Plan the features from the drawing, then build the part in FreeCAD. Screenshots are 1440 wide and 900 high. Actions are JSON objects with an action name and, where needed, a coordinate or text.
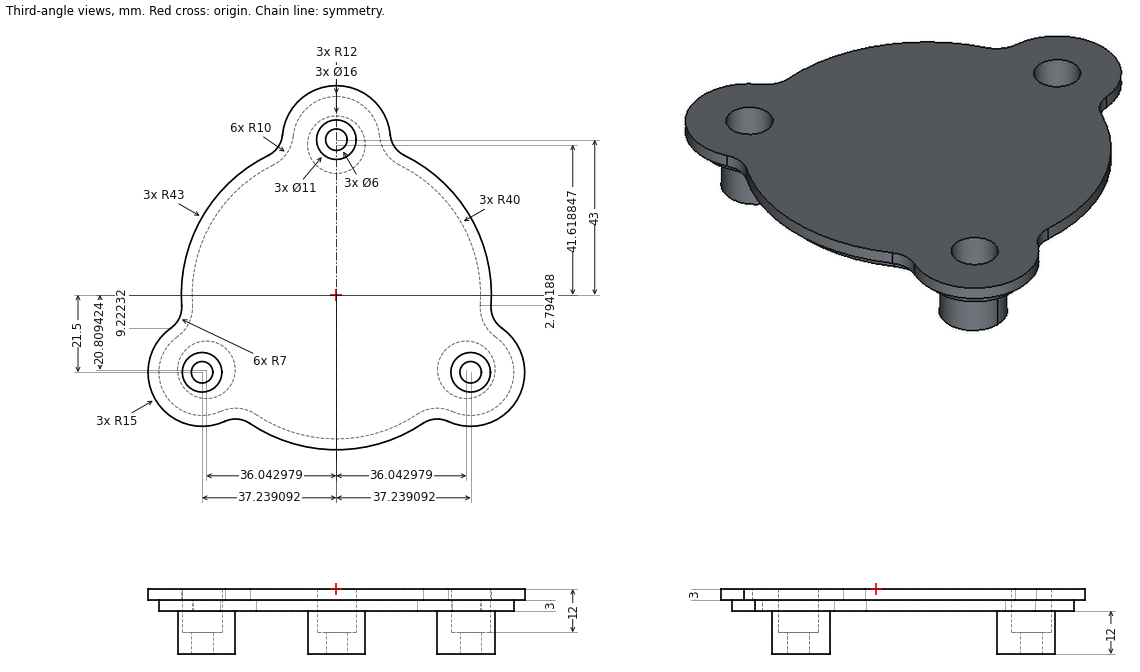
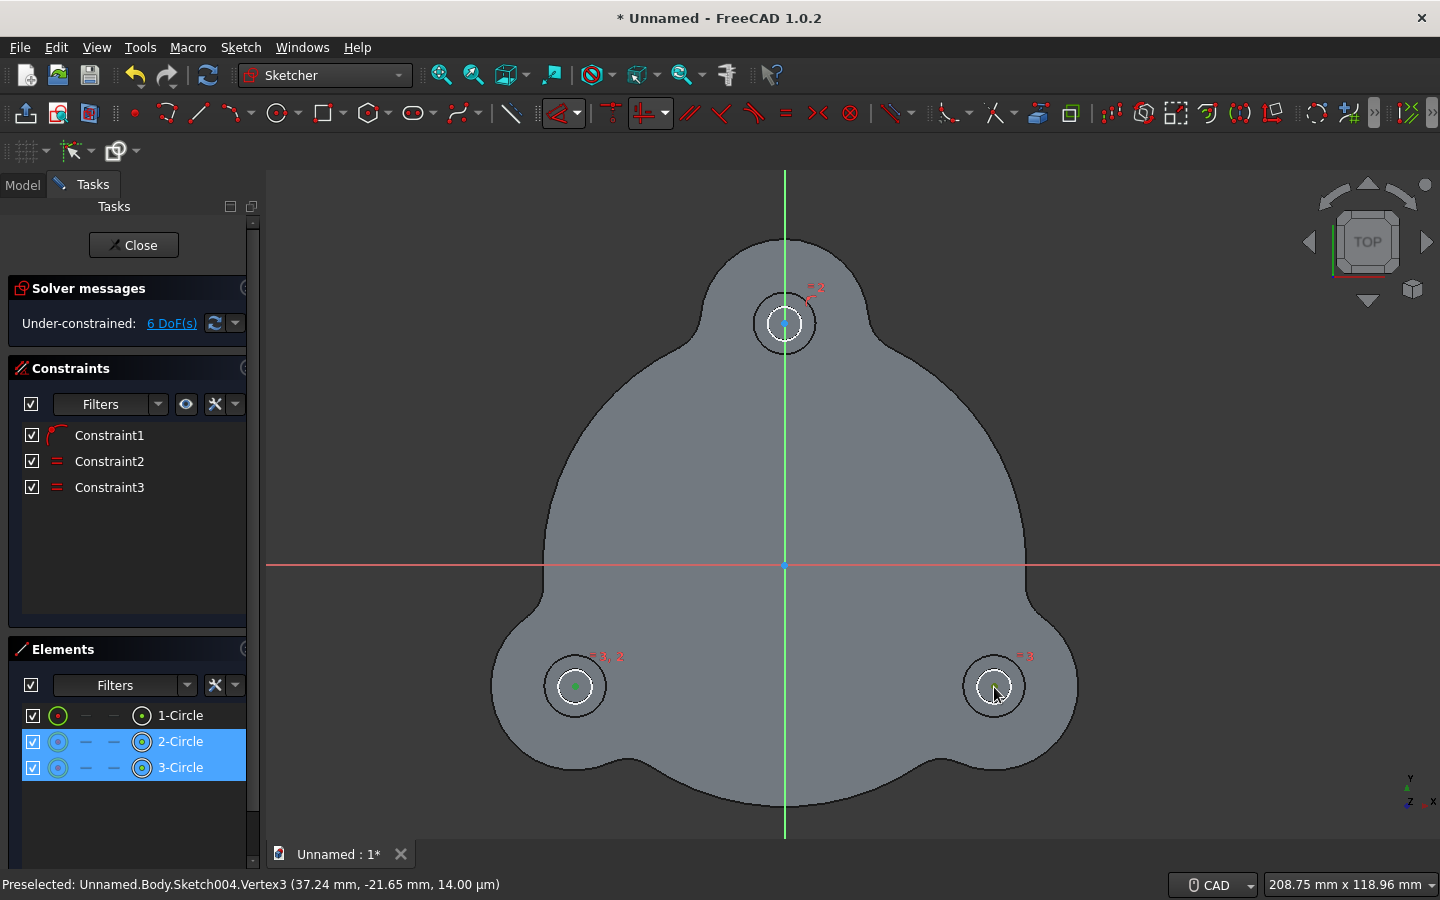
{"action": "key", "text": "h"}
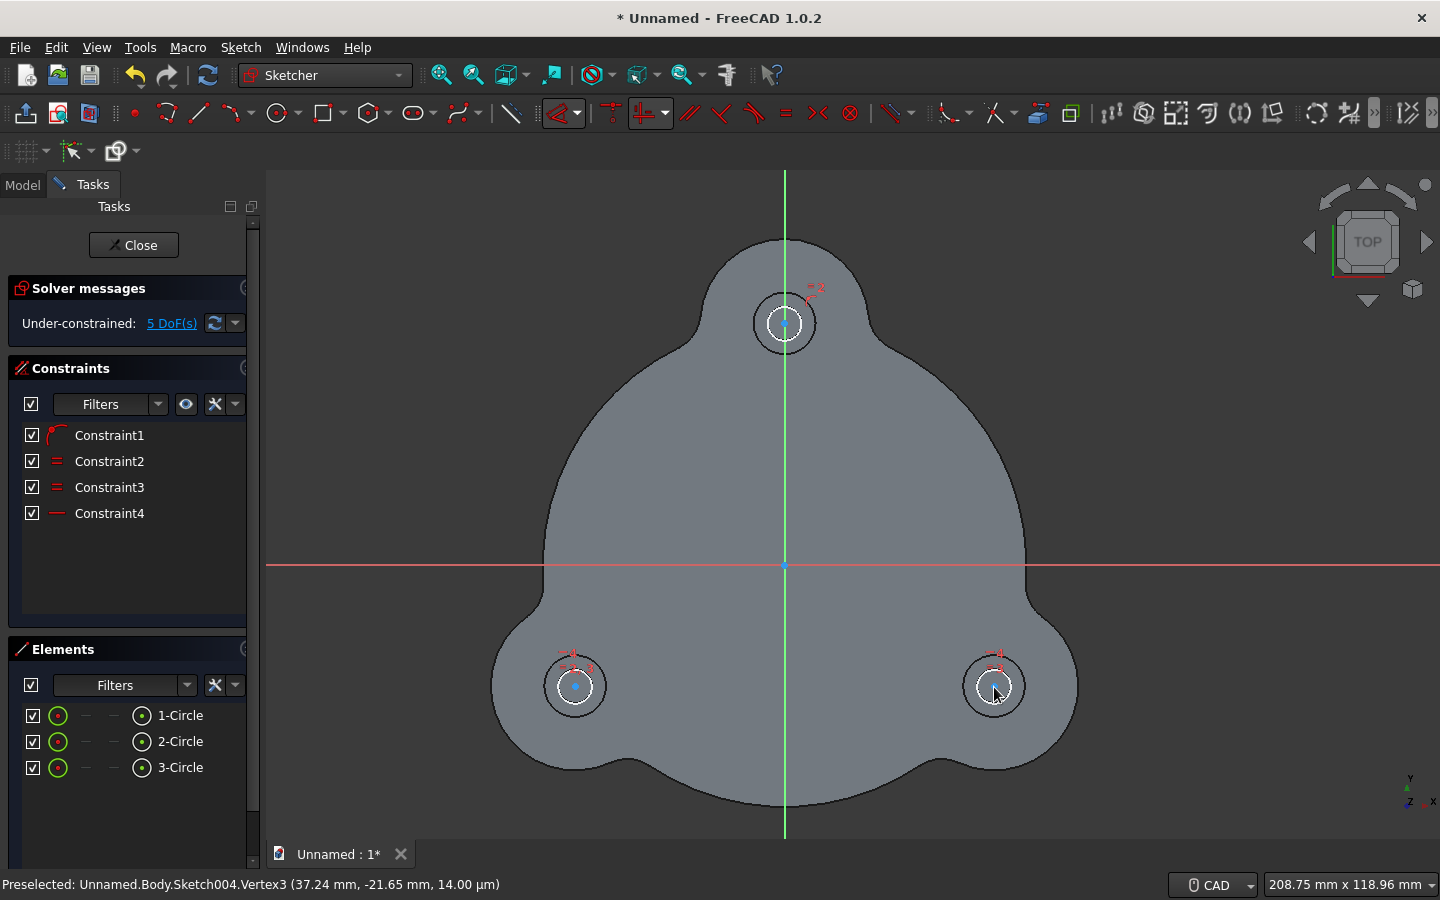
{"action": "left_click", "coordinate": [796, 312]}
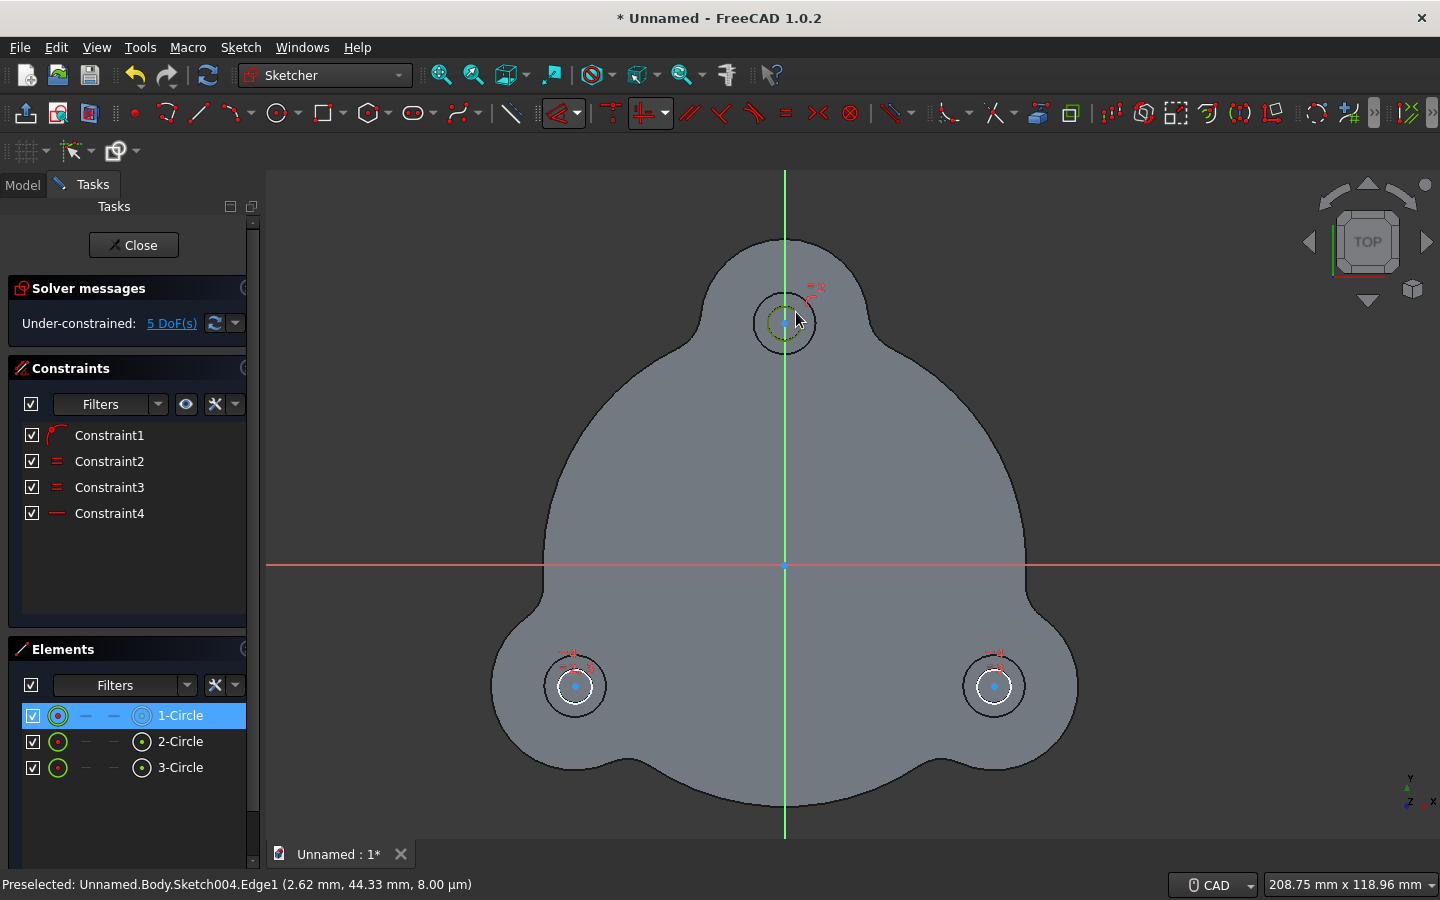
{"action": "key", "text": "k o"}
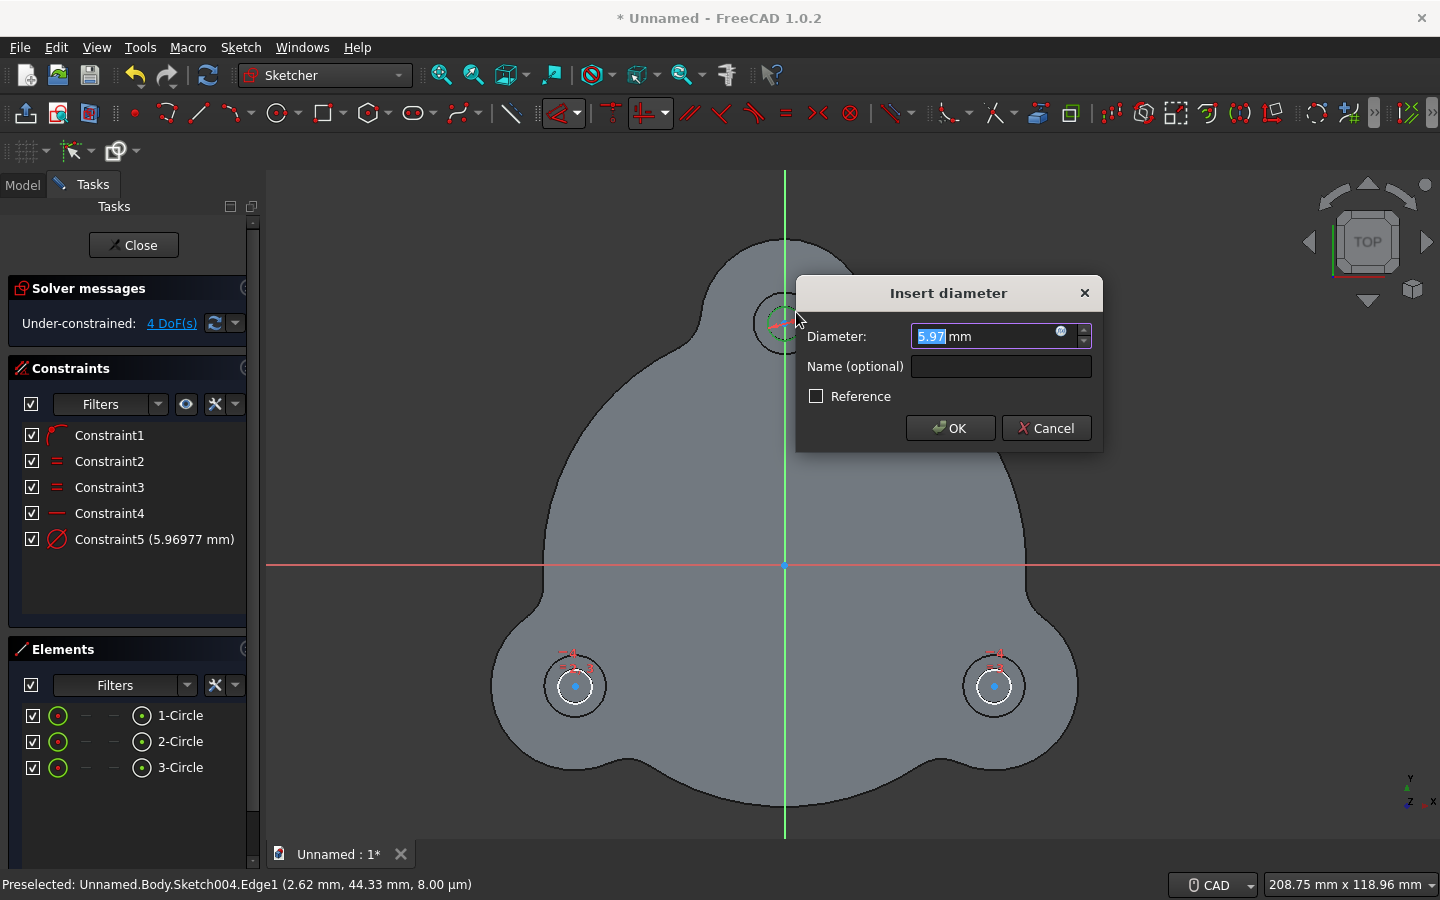
{"action": "type", "text": "6"}
{"action": "key", "text": "Return"}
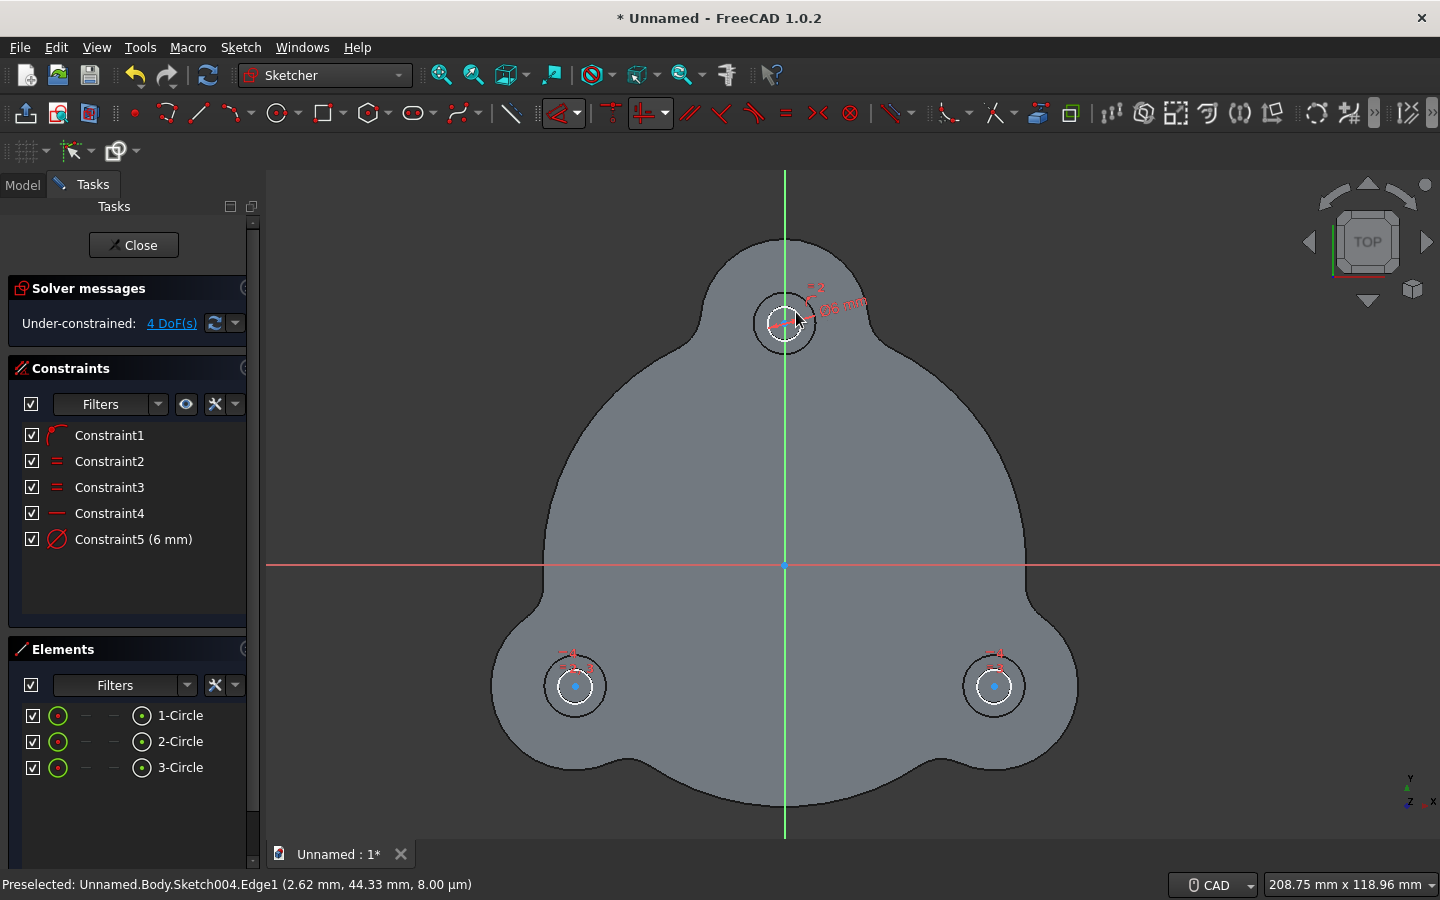
{"action": "left_click", "coordinate": [785, 324]}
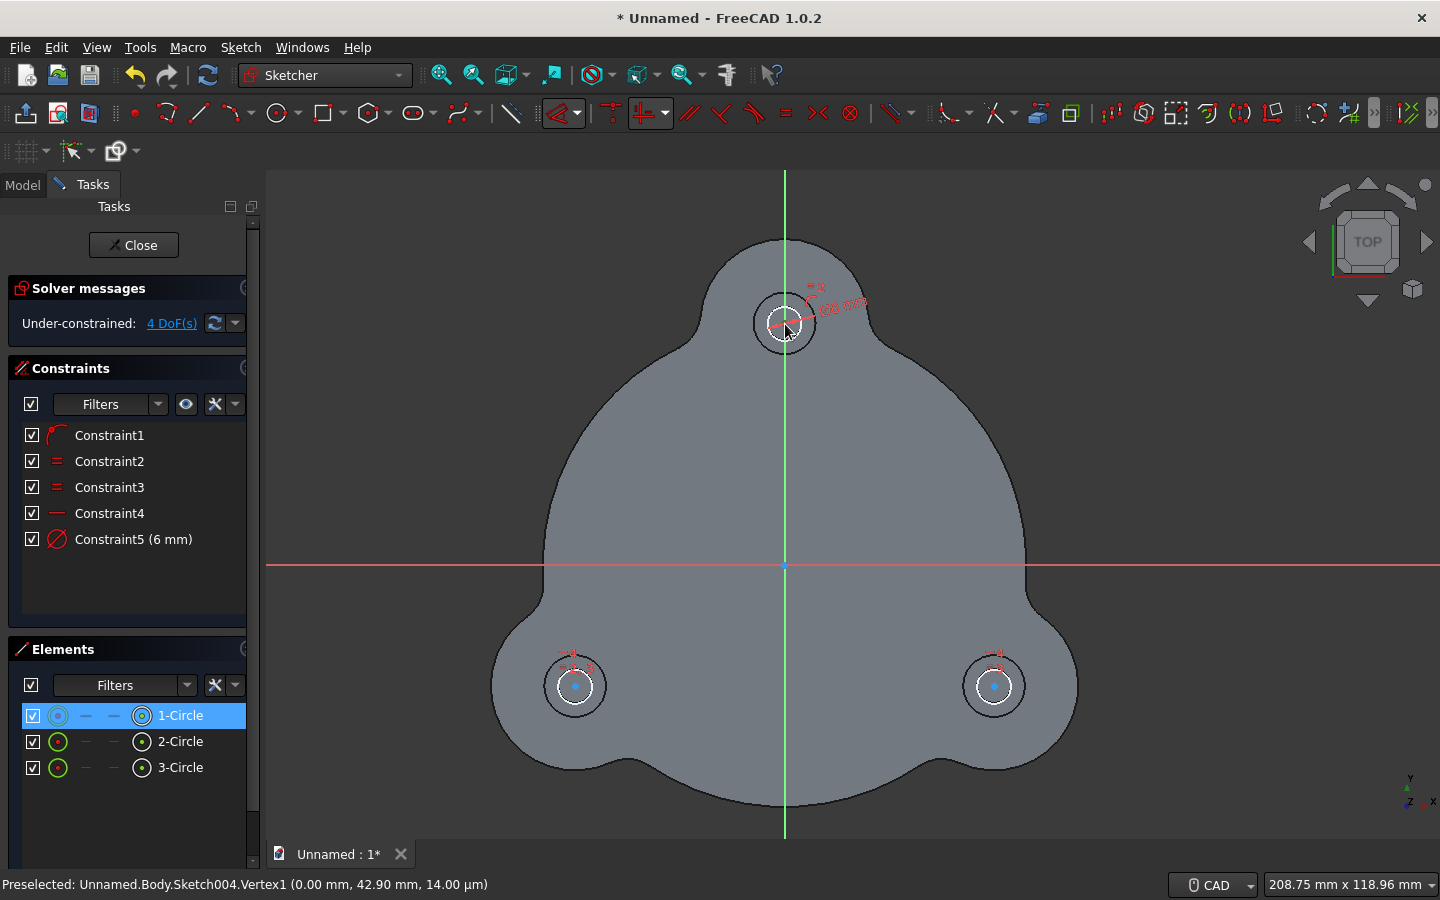
{"action": "left_click", "coordinate": [580, 114]}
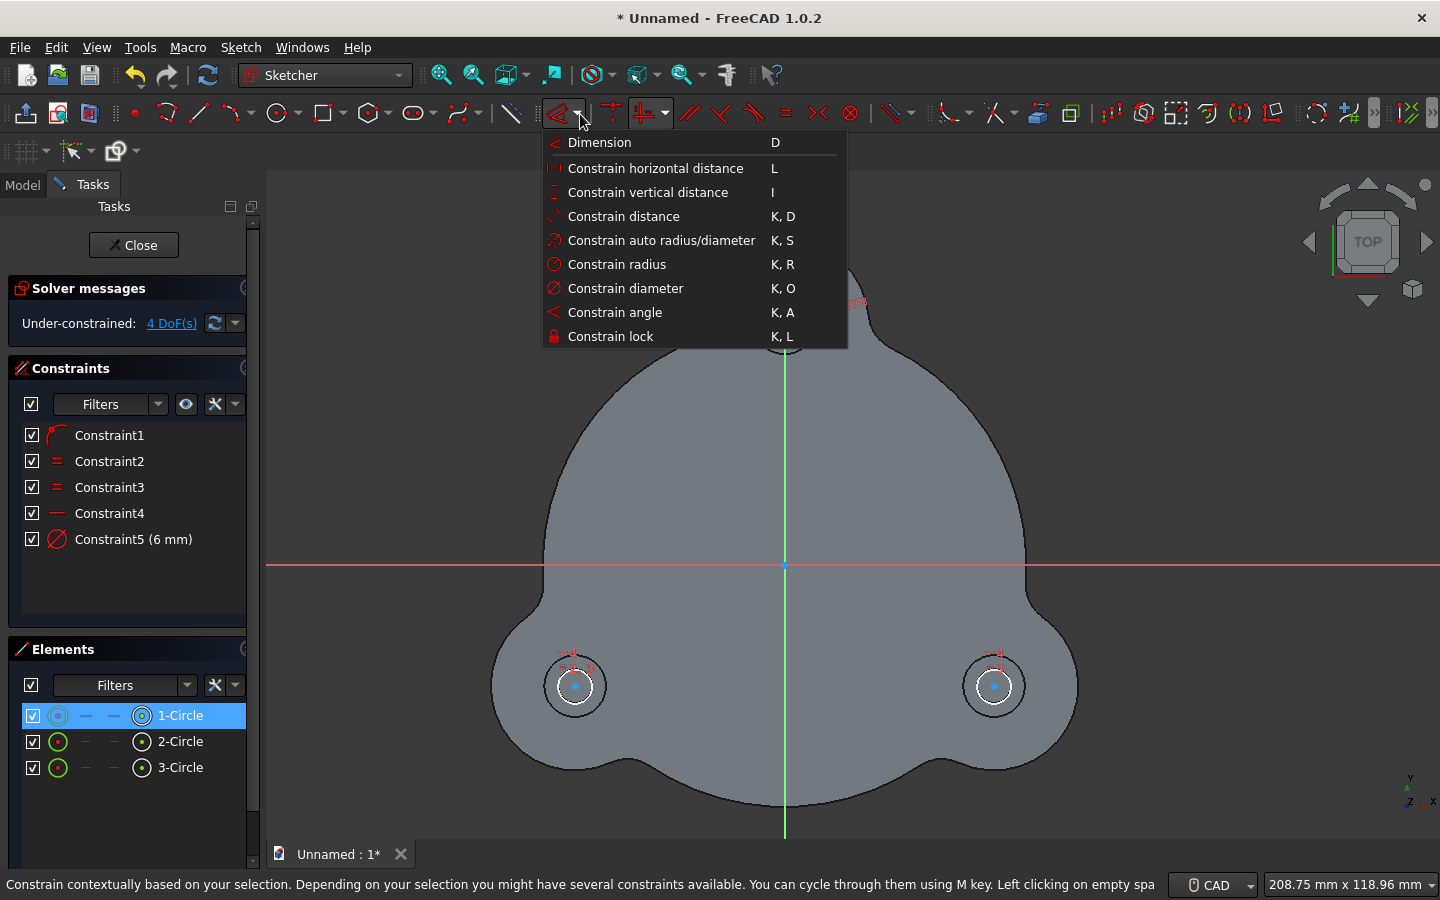
{"action": "left_click", "coordinate": [695, 192]}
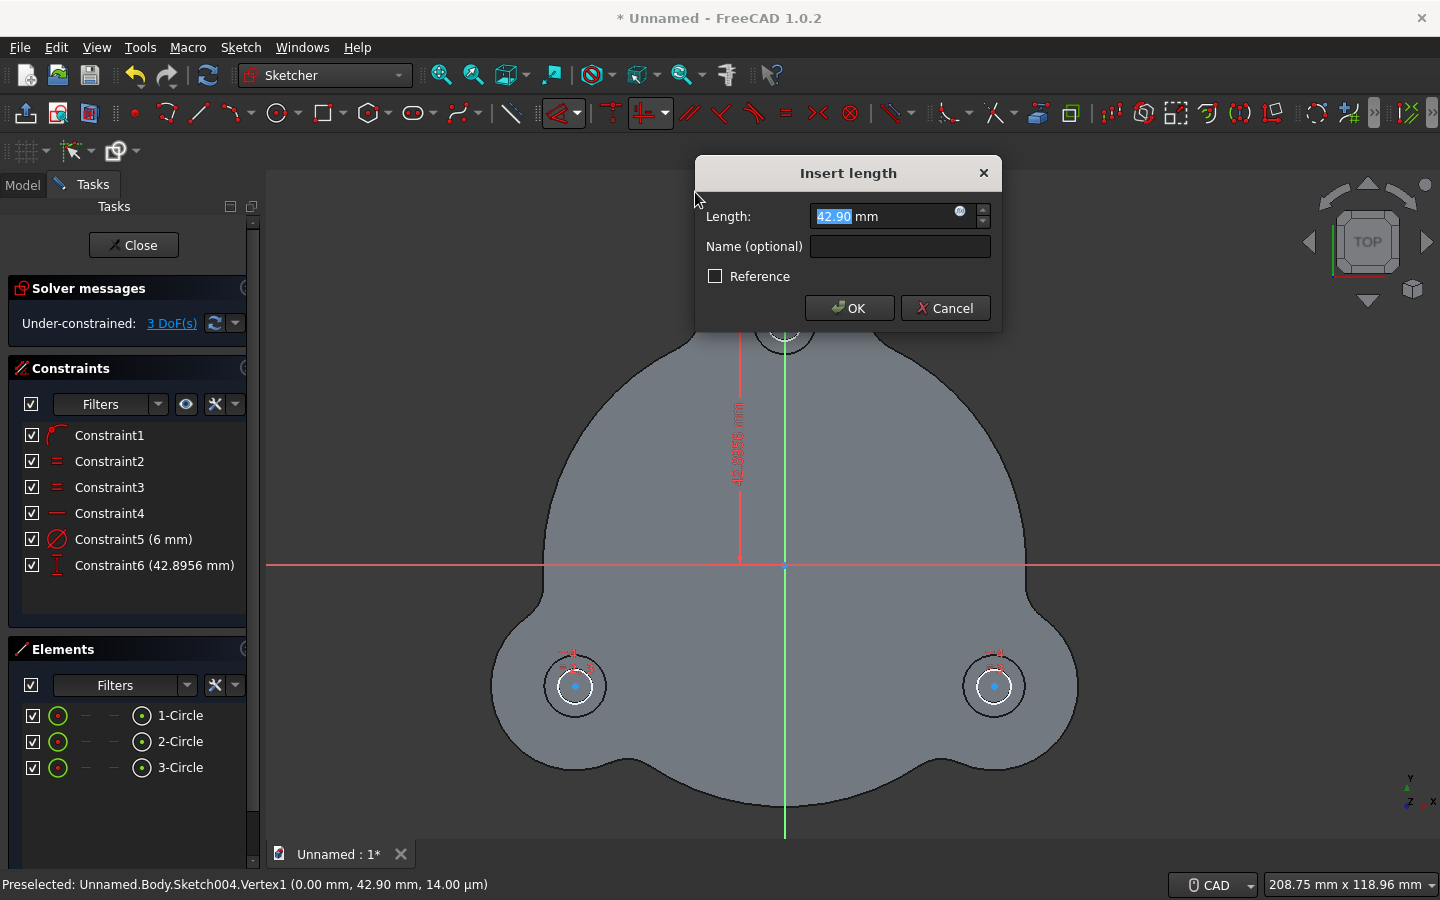
{"action": "type", "text": "43"}
{"action": "key", "text": "Return"}